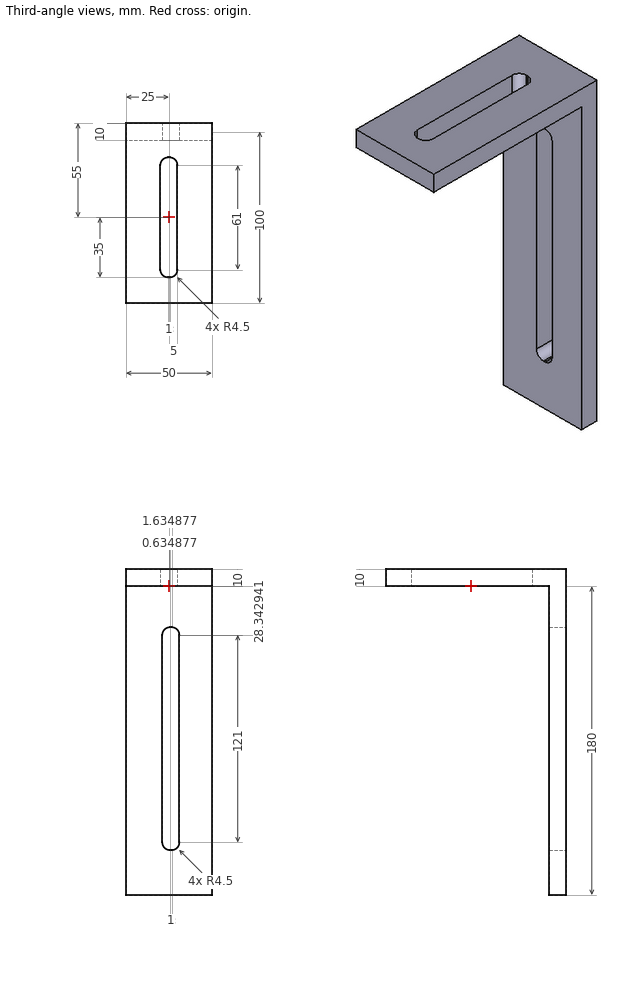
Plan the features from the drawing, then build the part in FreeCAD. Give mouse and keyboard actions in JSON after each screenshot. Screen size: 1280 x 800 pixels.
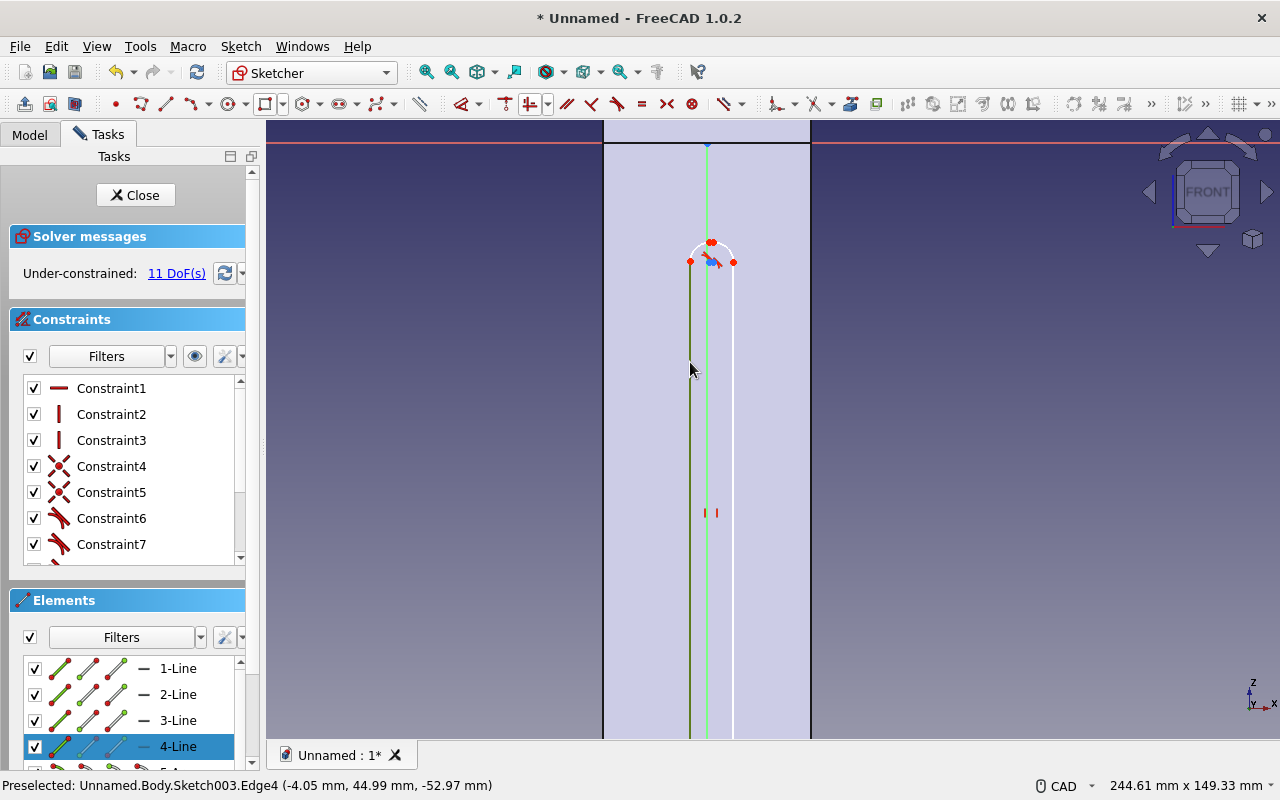
{"action": "scroll", "coordinate": [696, 248], "scroll_direction": "up", "scroll_amount": 2}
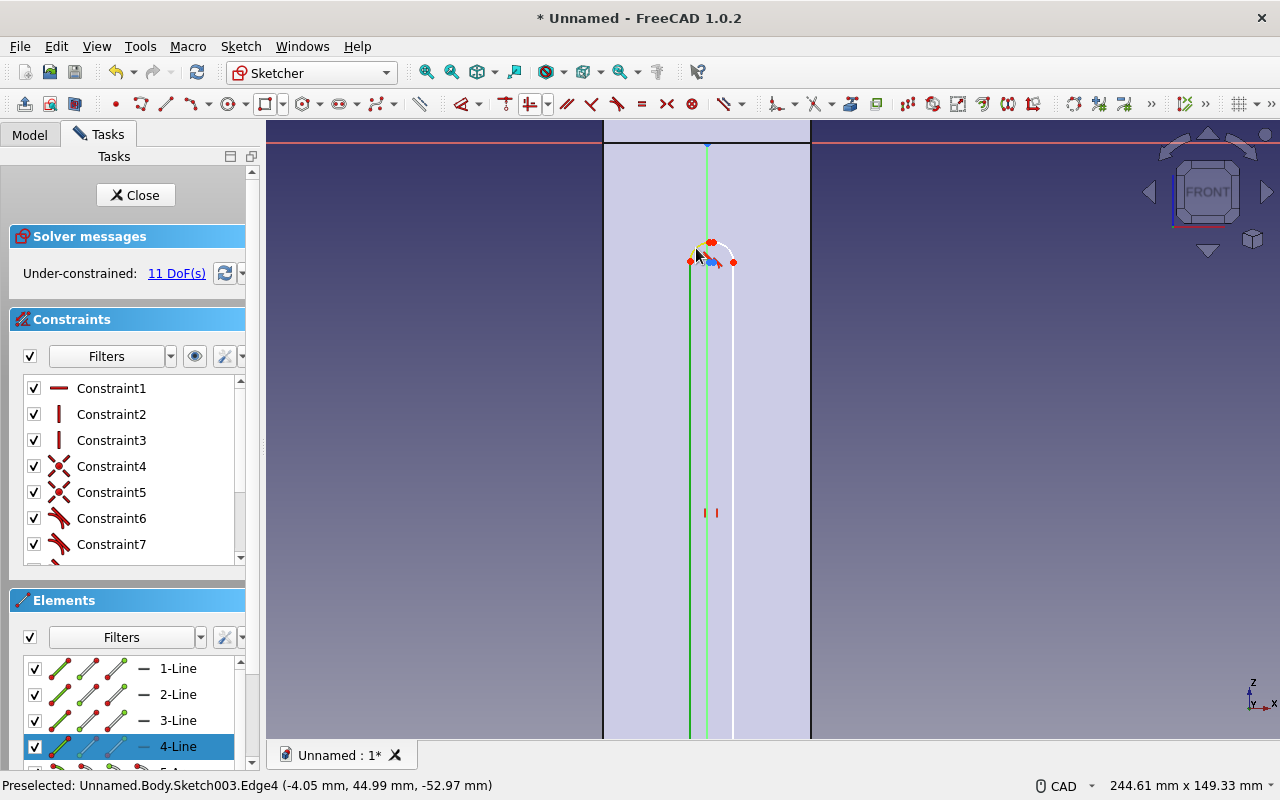
{"action": "left_click", "coordinate": [696, 248]}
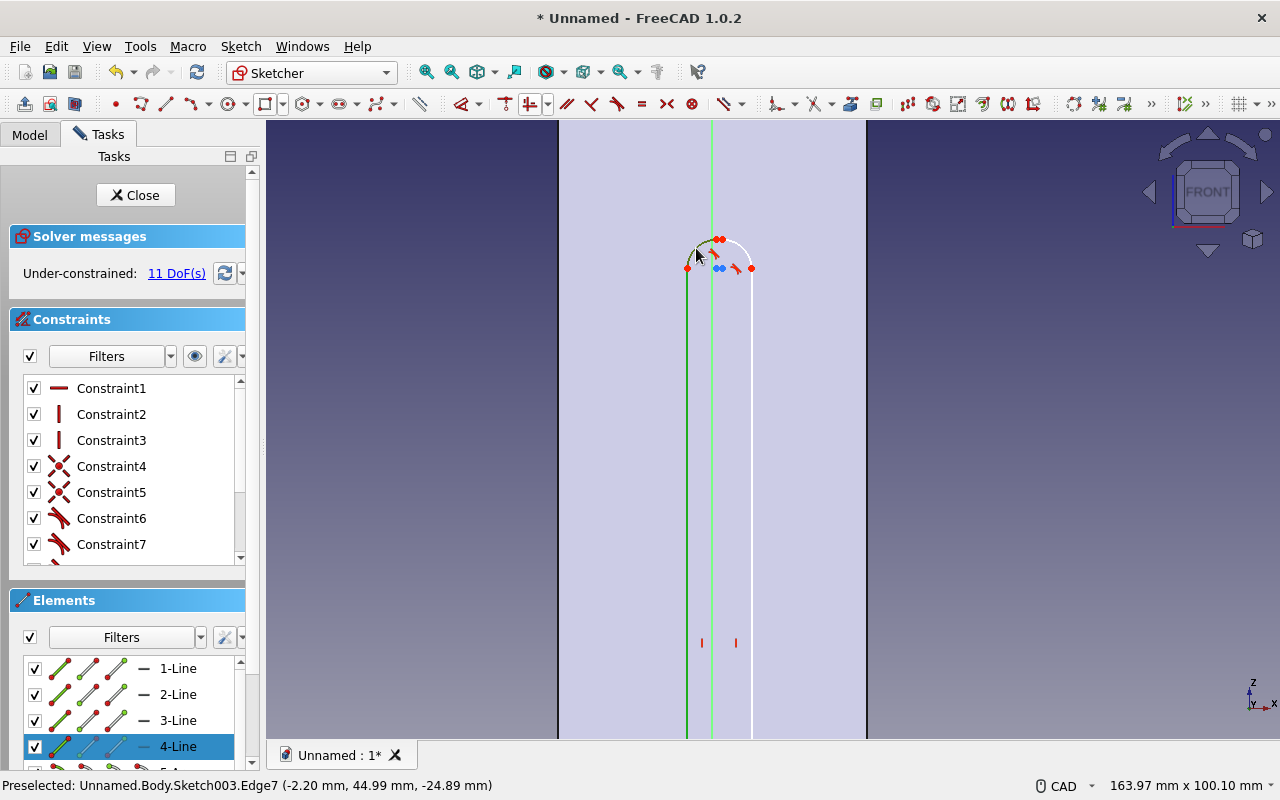
{"action": "left_click", "coordinate": [617, 104]}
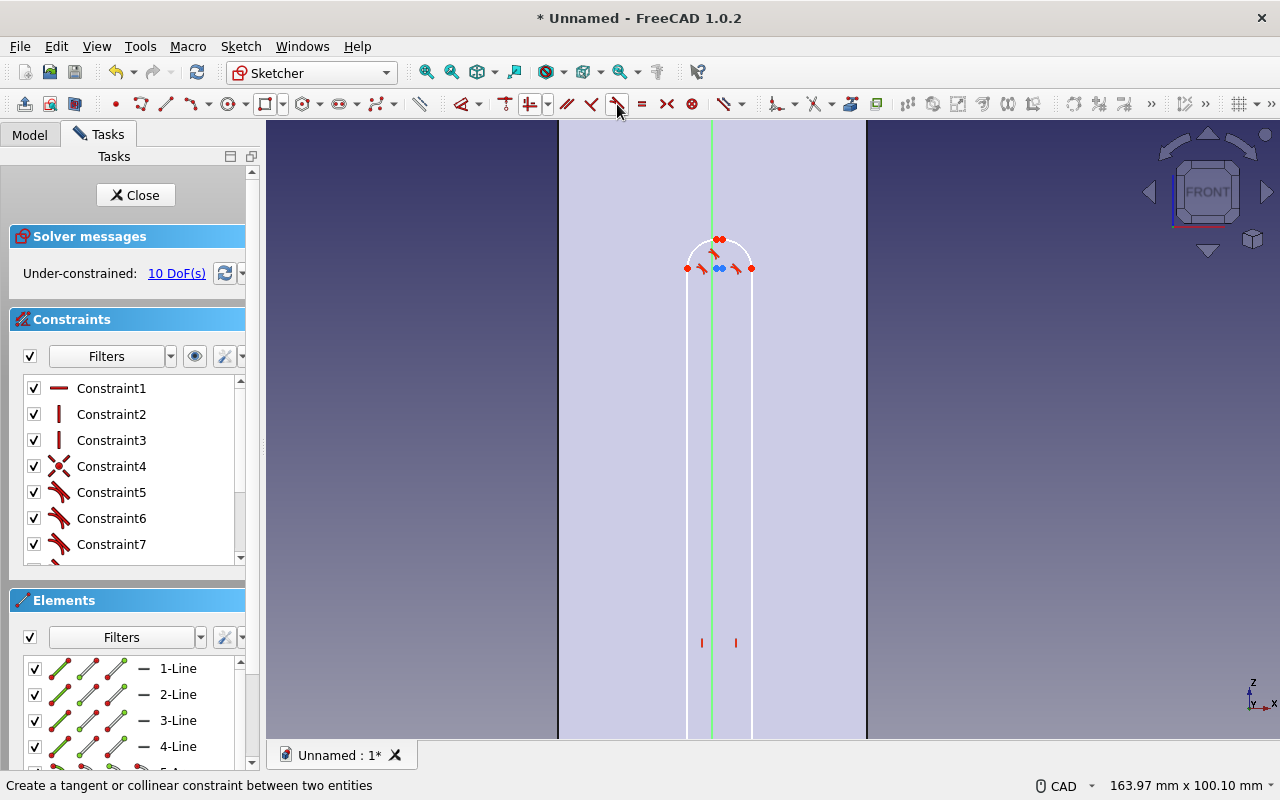
{"action": "left_click", "coordinate": [687, 493]}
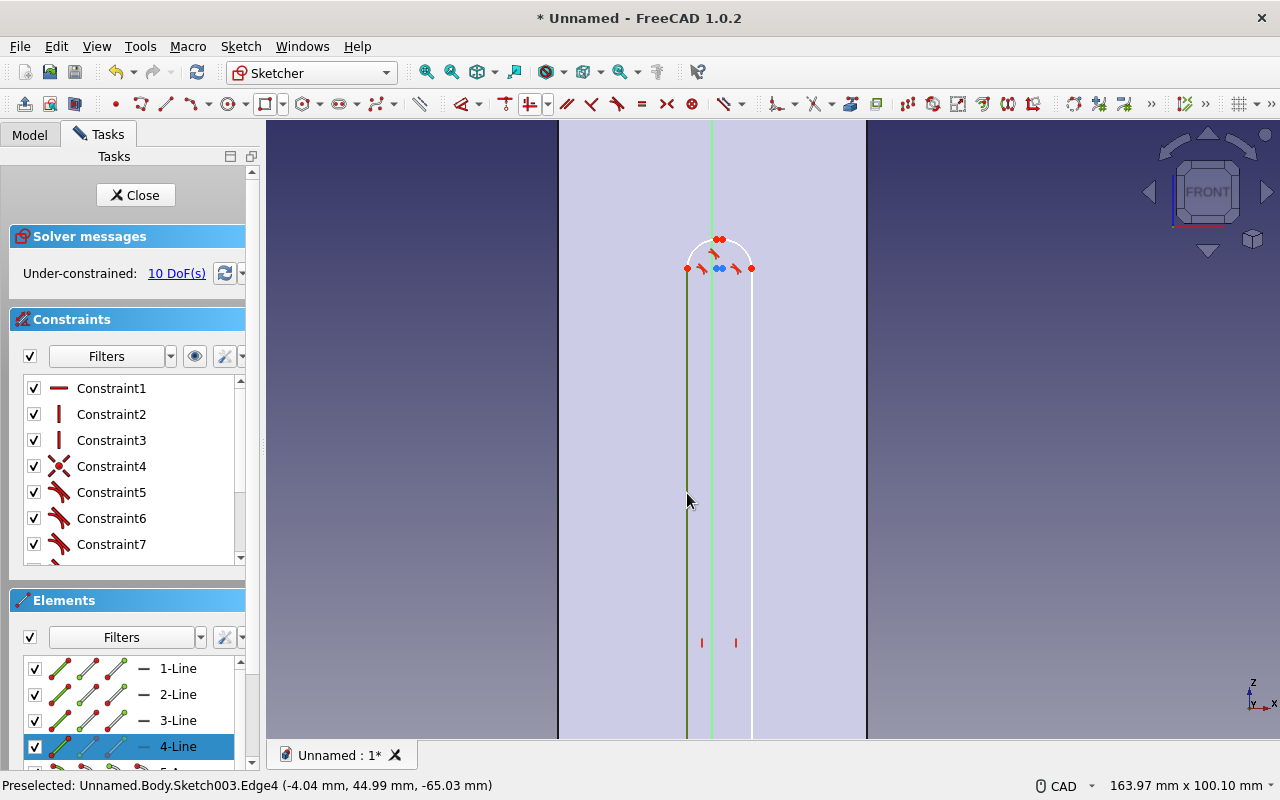
{"action": "scroll", "coordinate": [692, 317], "scroll_direction": "down", "scroll_amount": 4}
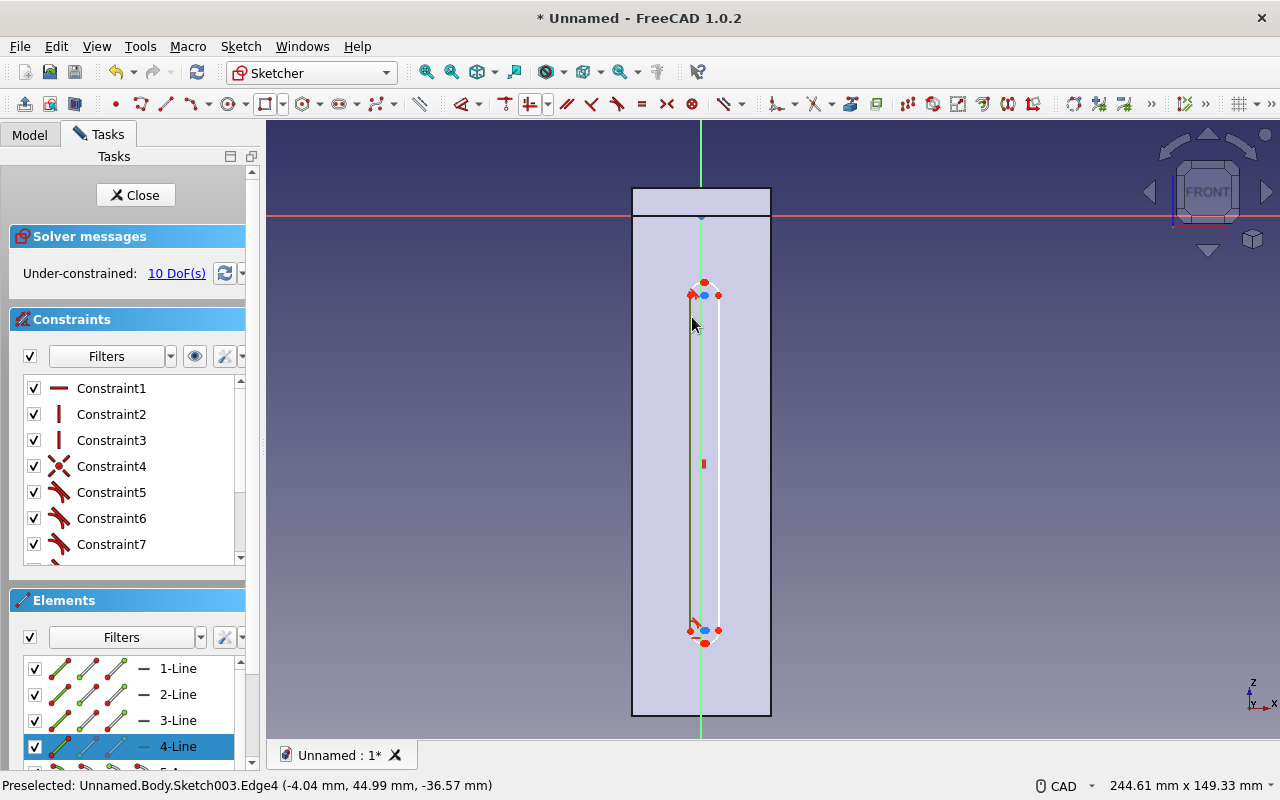
{"action": "scroll", "coordinate": [692, 637], "scroll_direction": "up", "scroll_amount": 5}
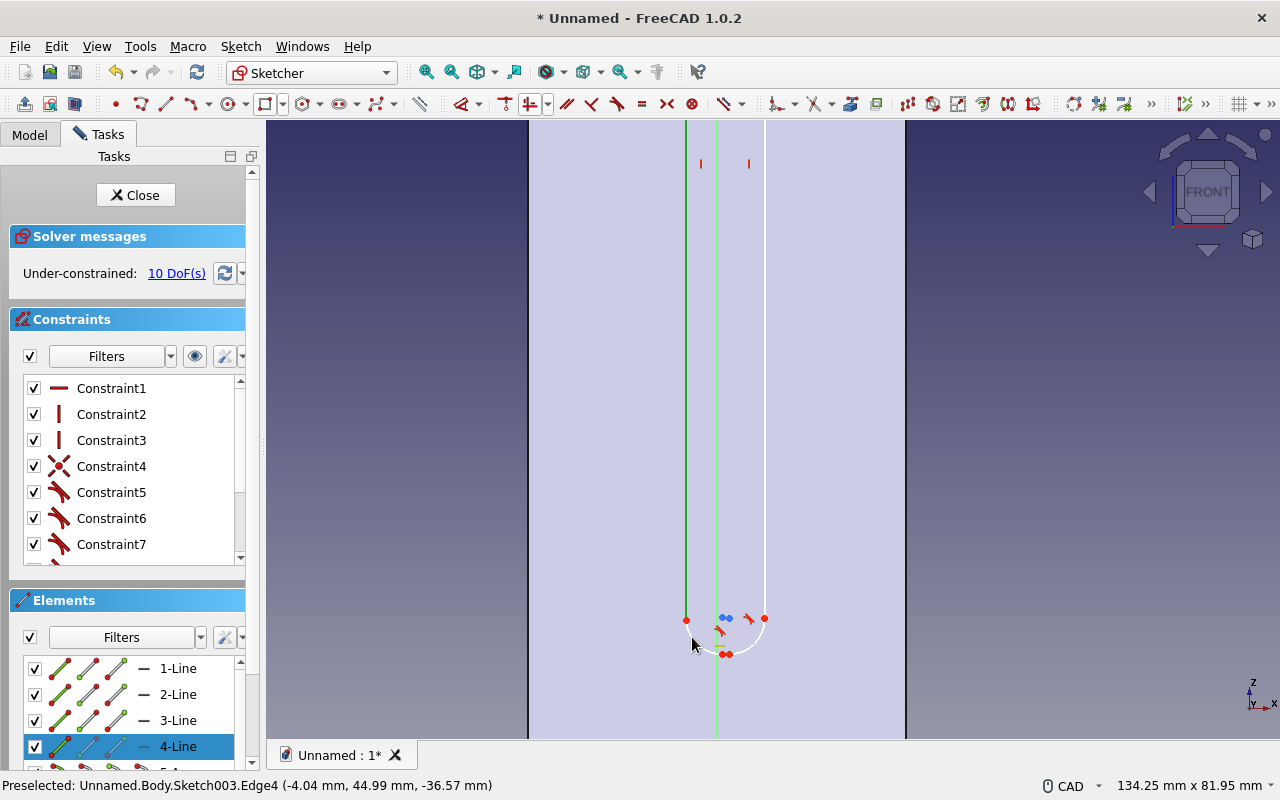
{"action": "left_click", "coordinate": [691, 636]}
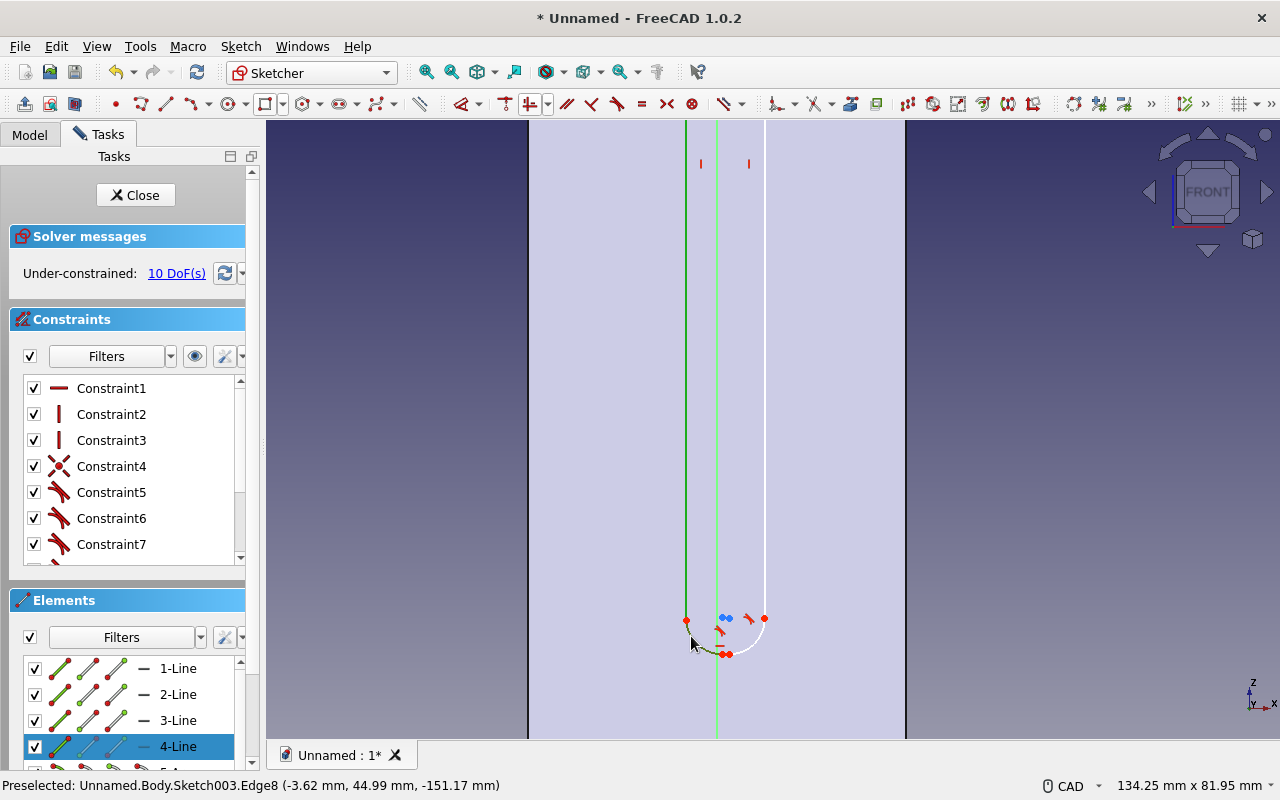
{"action": "left_click", "coordinate": [617, 104]}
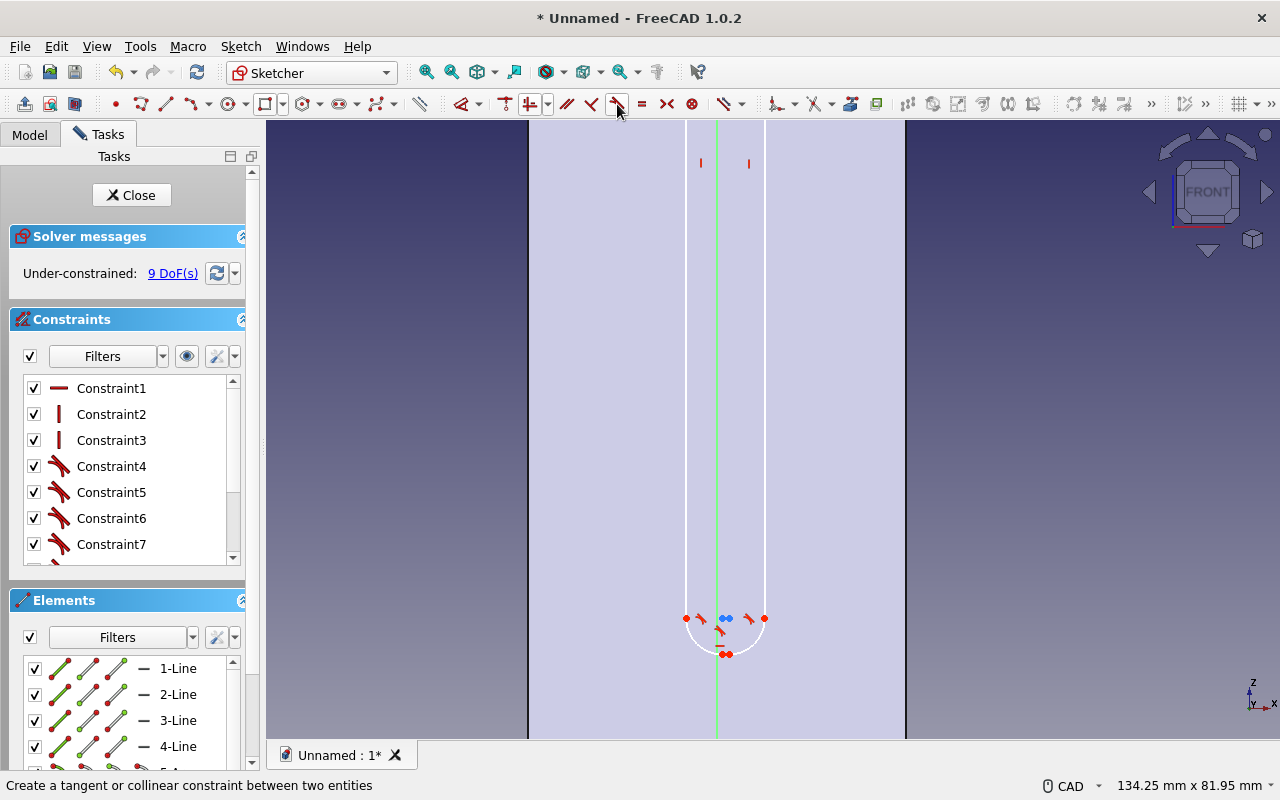
{"action": "left_click", "coordinate": [745, 651]}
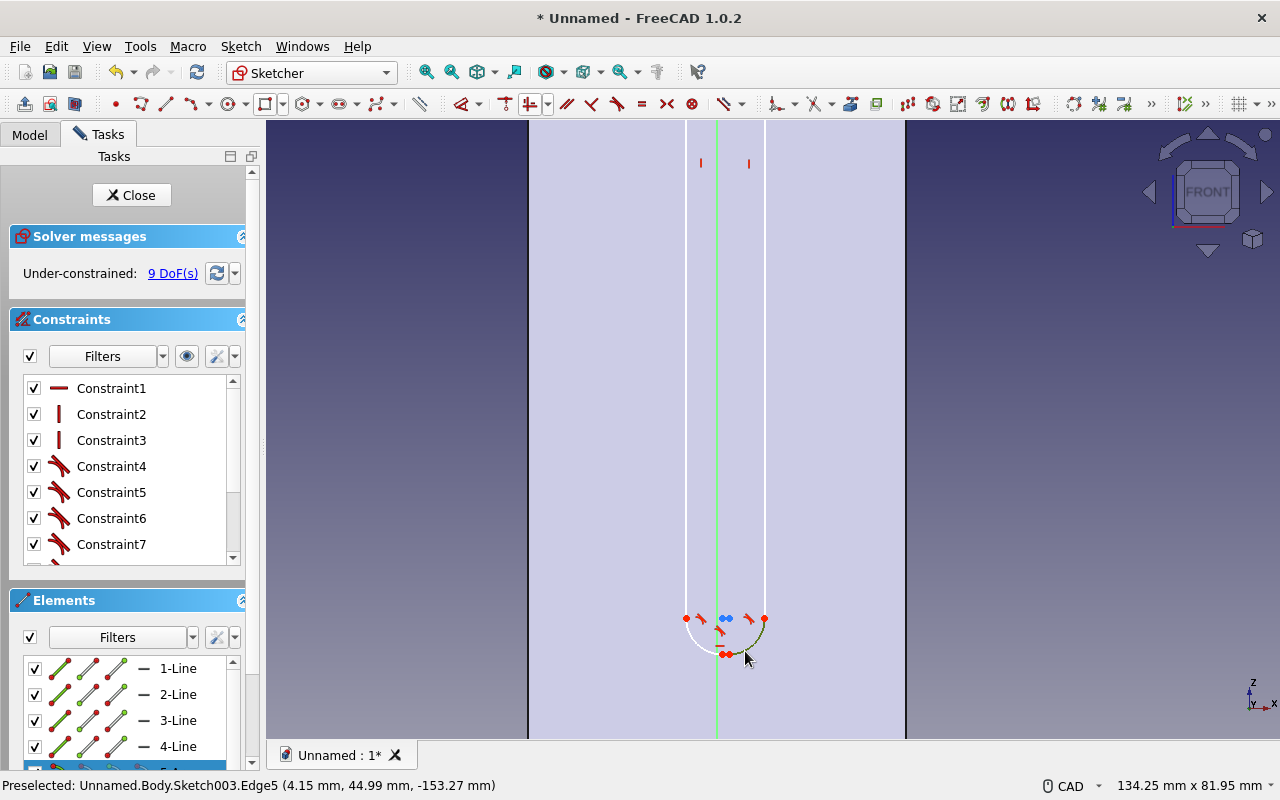
{"action": "scroll", "coordinate": [692, 637], "scroll_direction": "down", "scroll_amount": 5}